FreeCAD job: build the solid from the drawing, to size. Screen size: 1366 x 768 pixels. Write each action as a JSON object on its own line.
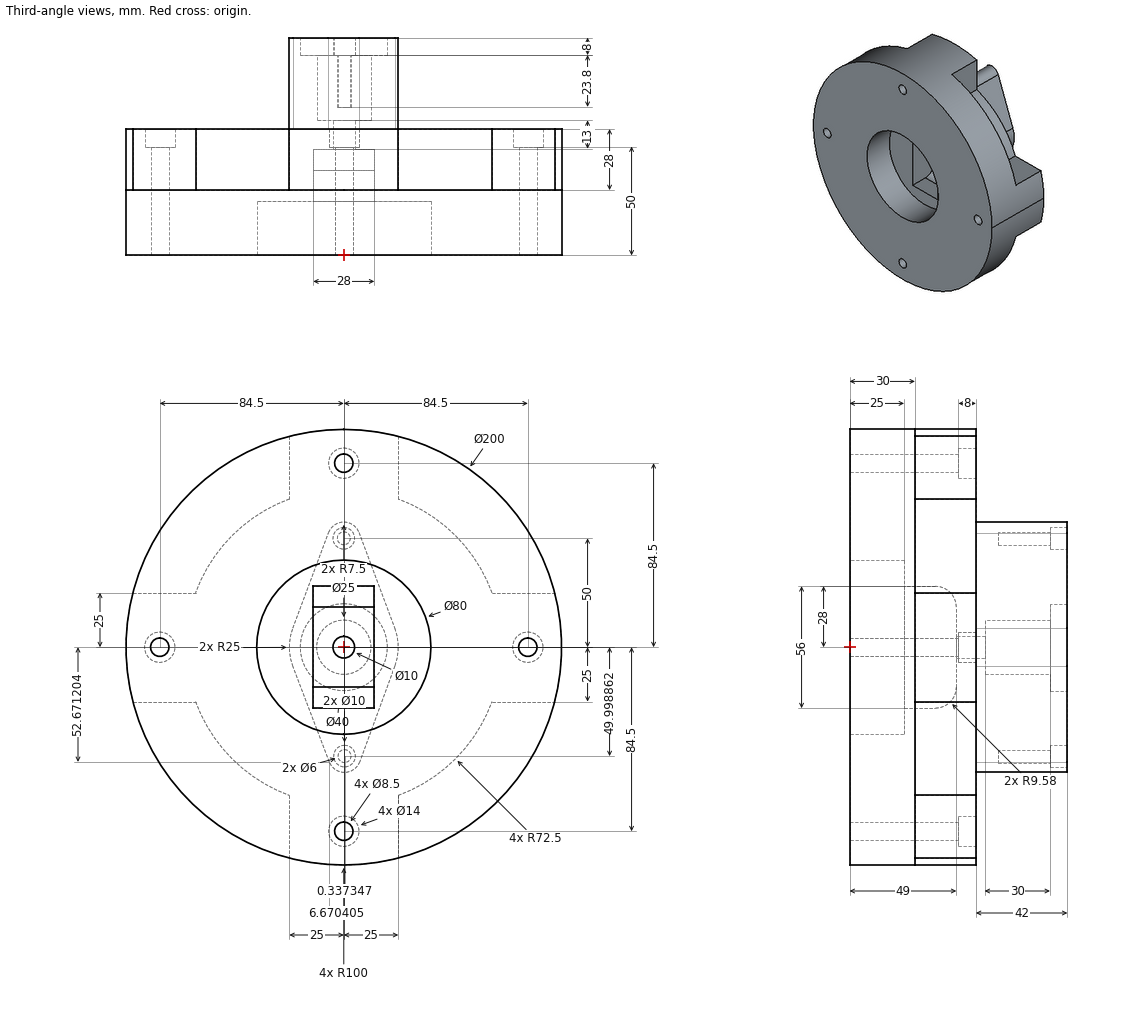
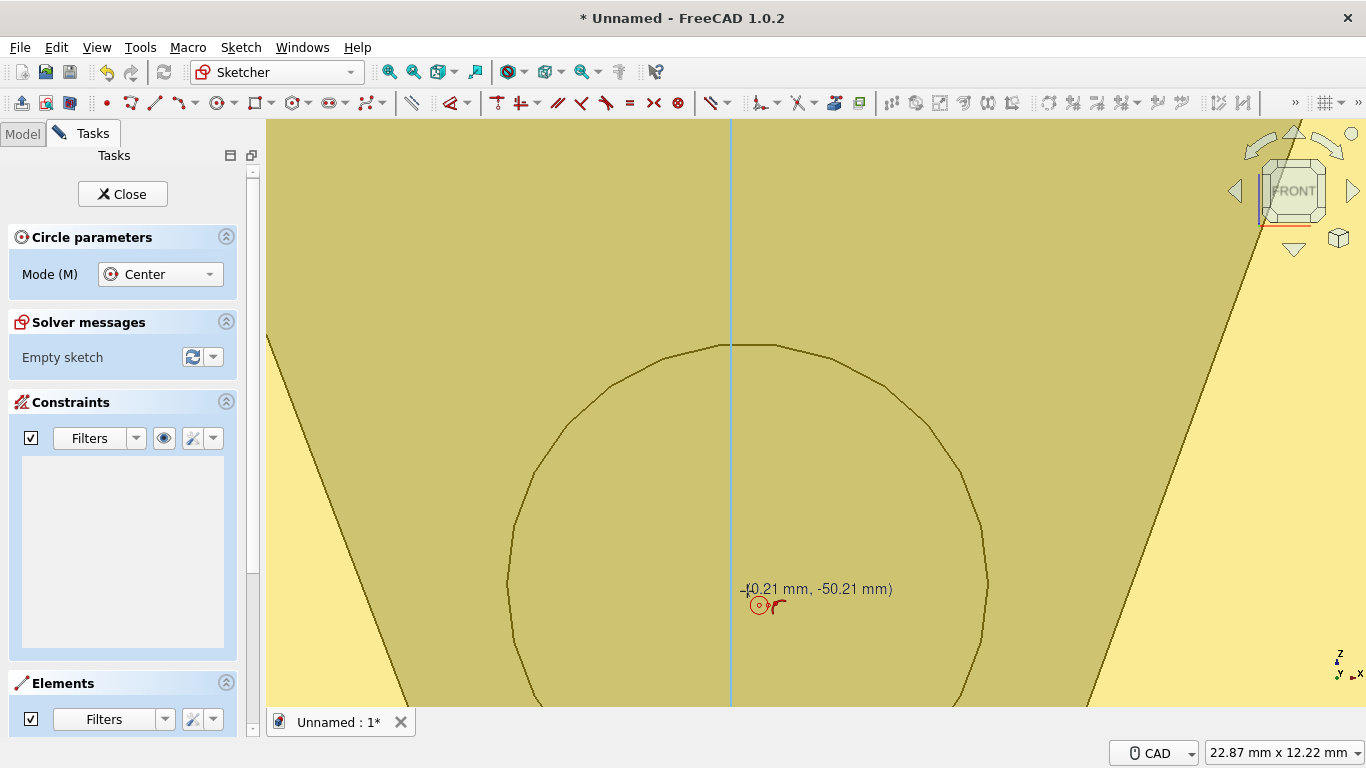
{"action": "left_click", "coordinate": [748, 584]}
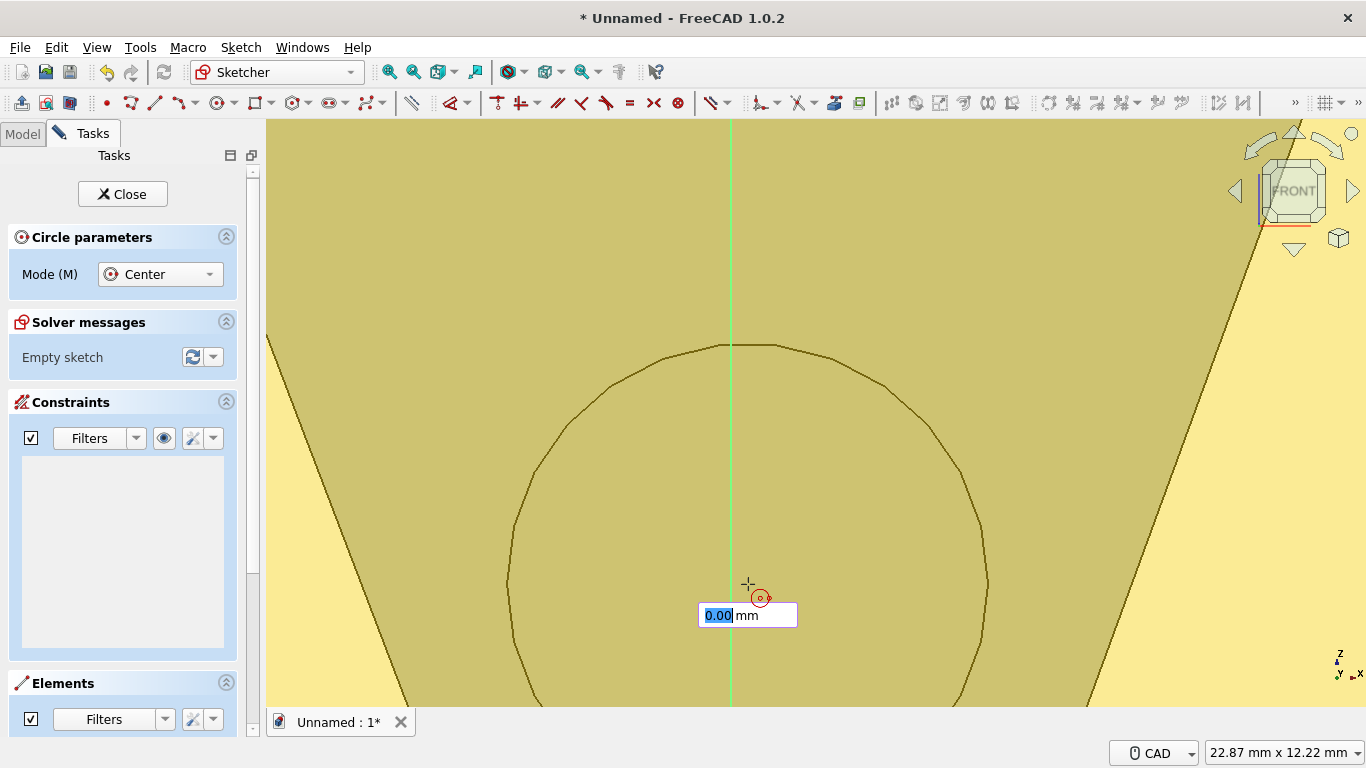
{"action": "scroll", "coordinate": [748, 592], "scroll_direction": "down", "scroll_amount": 13}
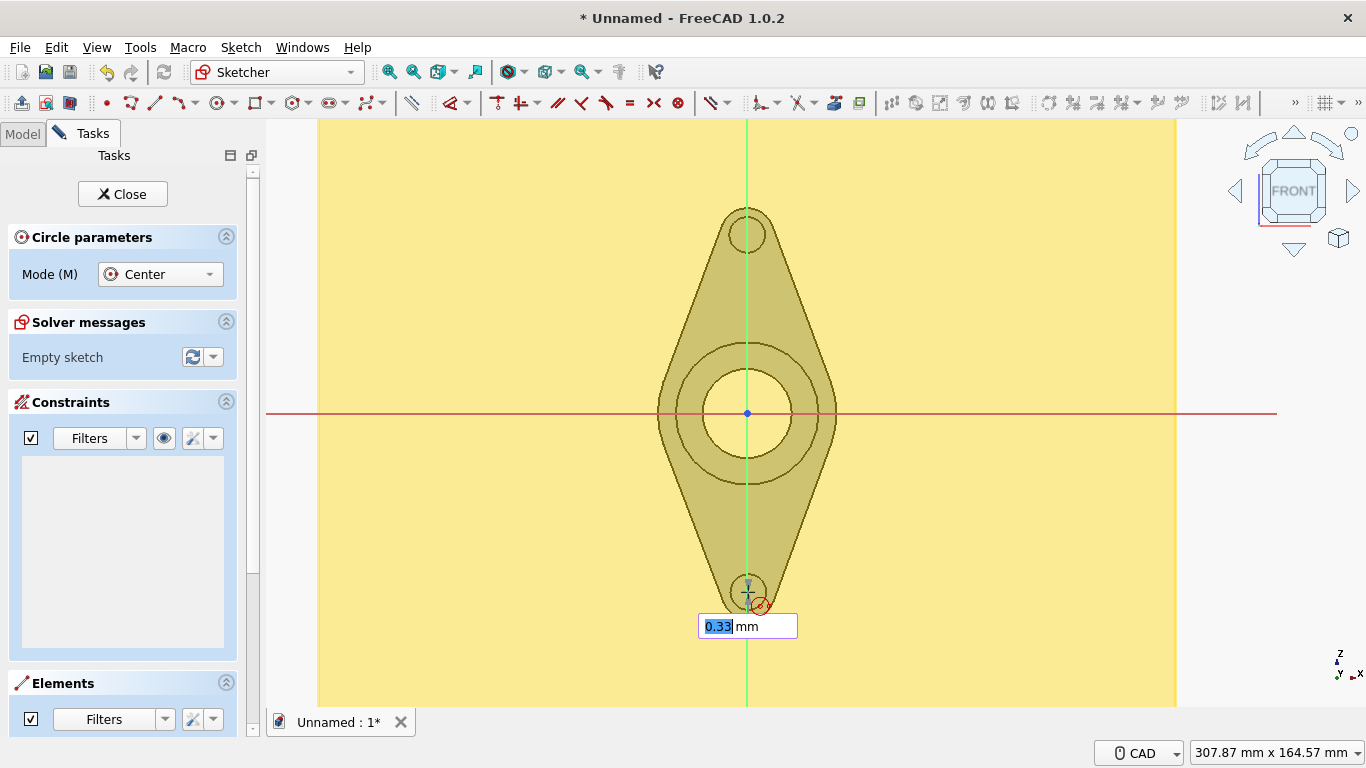
{"action": "scroll", "coordinate": [756, 585], "scroll_direction": "up", "scroll_amount": 3}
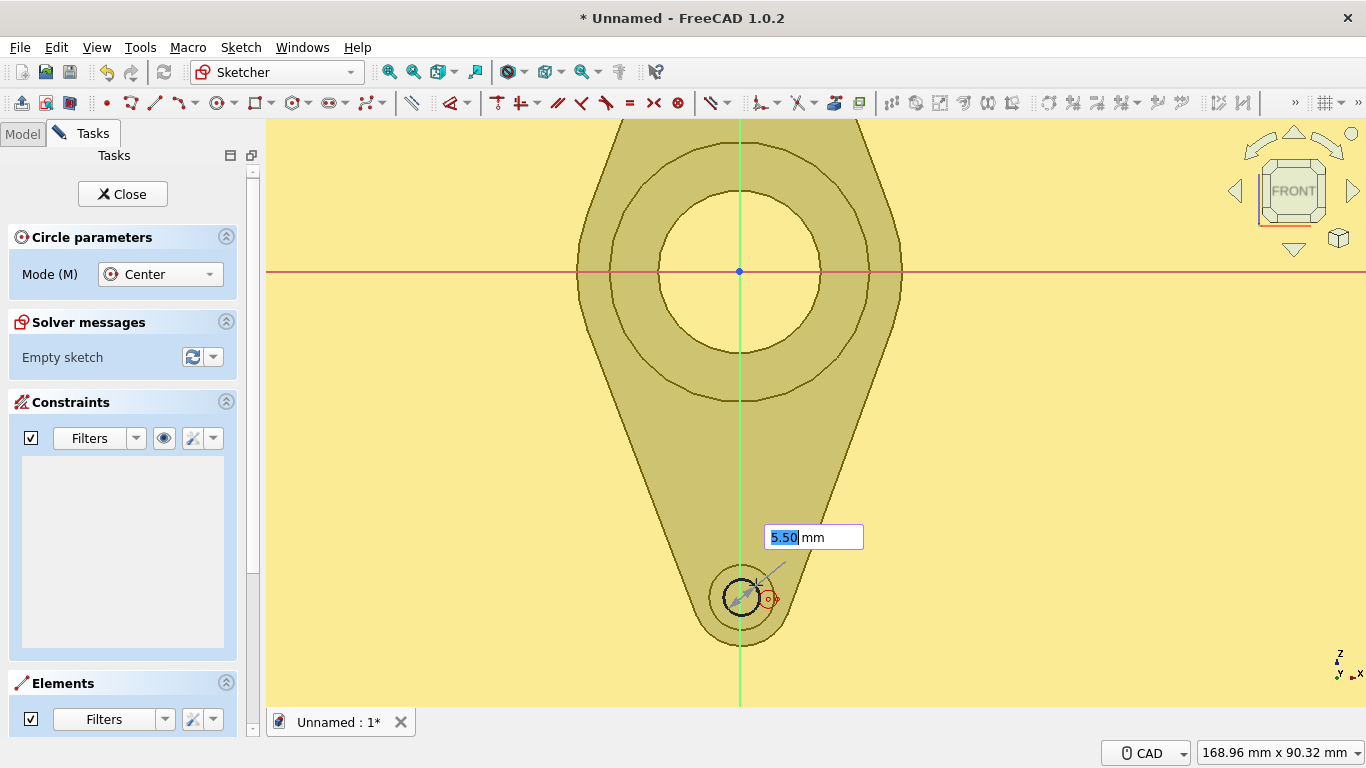
{"action": "left_click", "coordinate": [756, 584]}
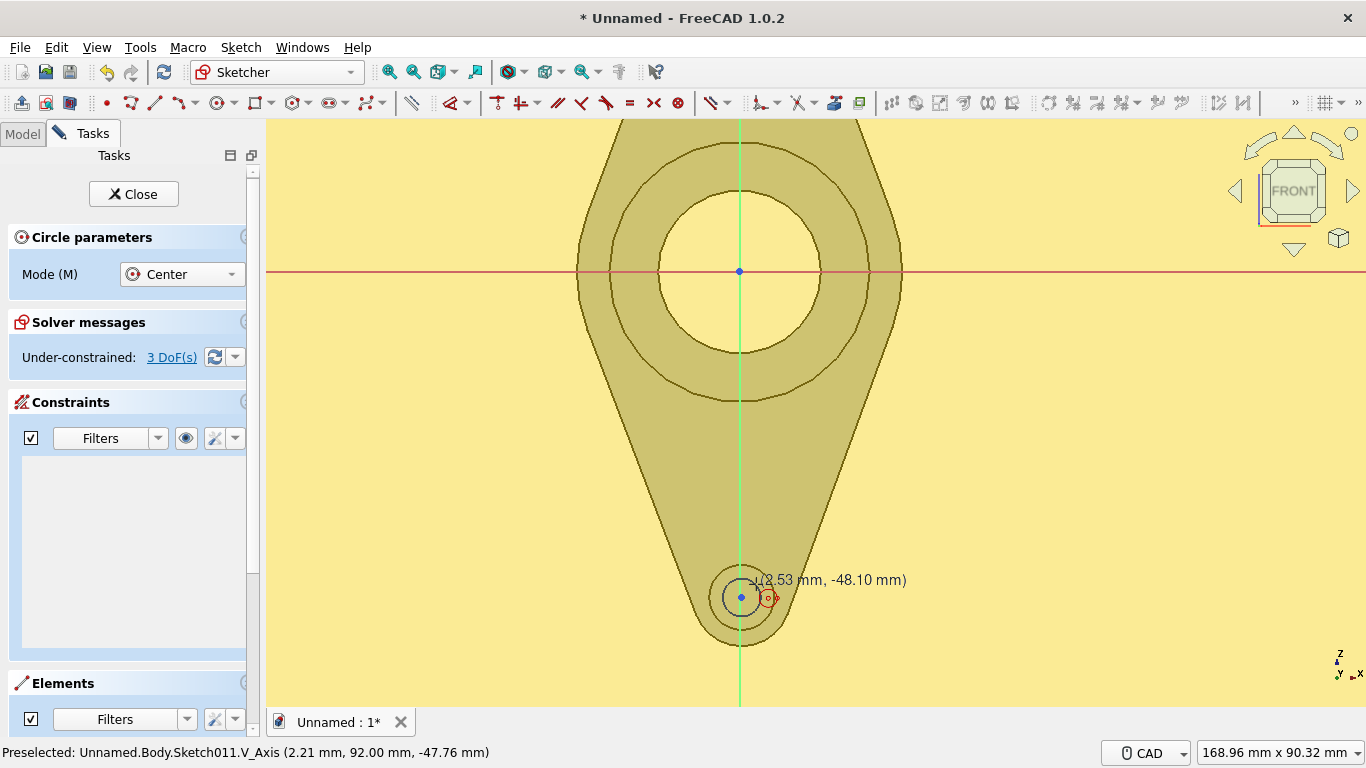
{"action": "scroll", "coordinate": [756, 585], "scroll_direction": "down", "scroll_amount": 3}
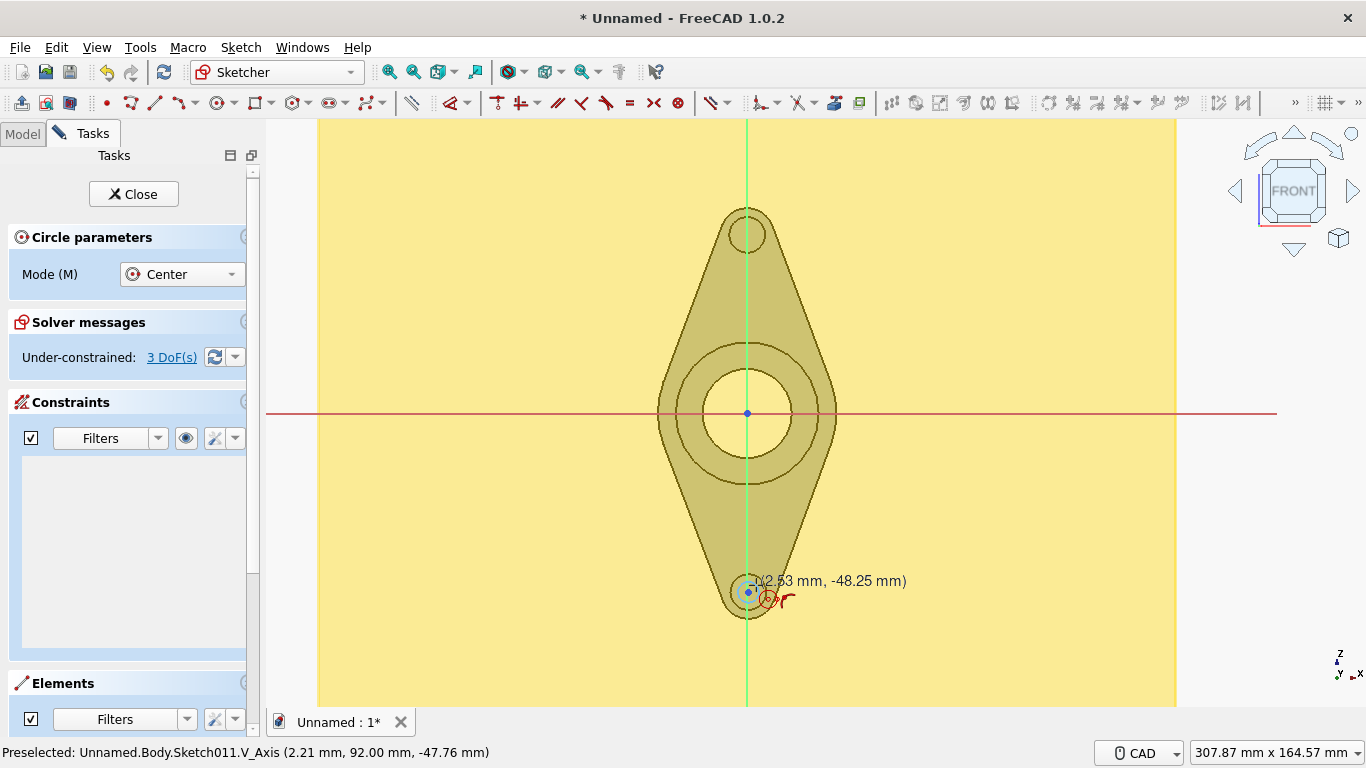
{"action": "scroll", "coordinate": [747, 235], "scroll_direction": "up", "scroll_amount": 4}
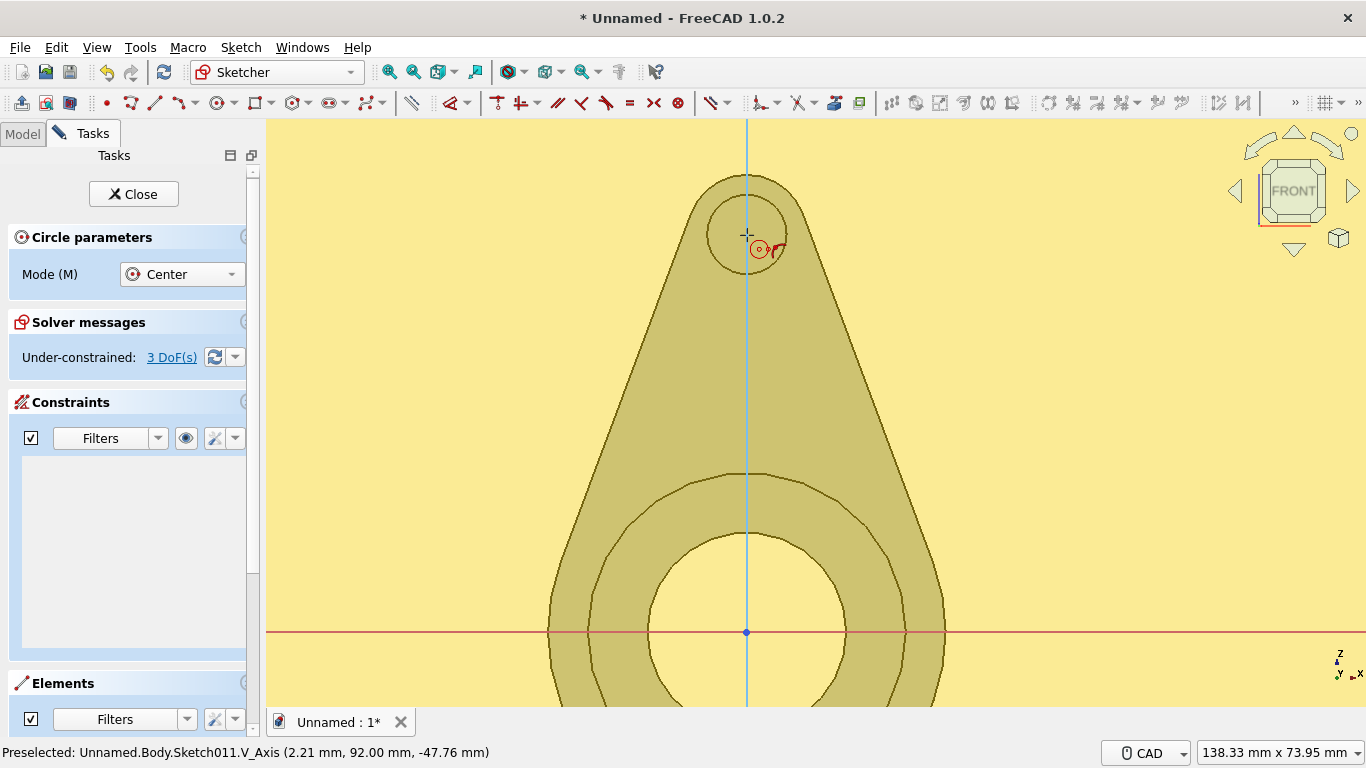
{"action": "left_click", "coordinate": [747, 234]}
{"action": "left_click", "coordinate": [764, 218]}
{"action": "key", "text": "Escape"}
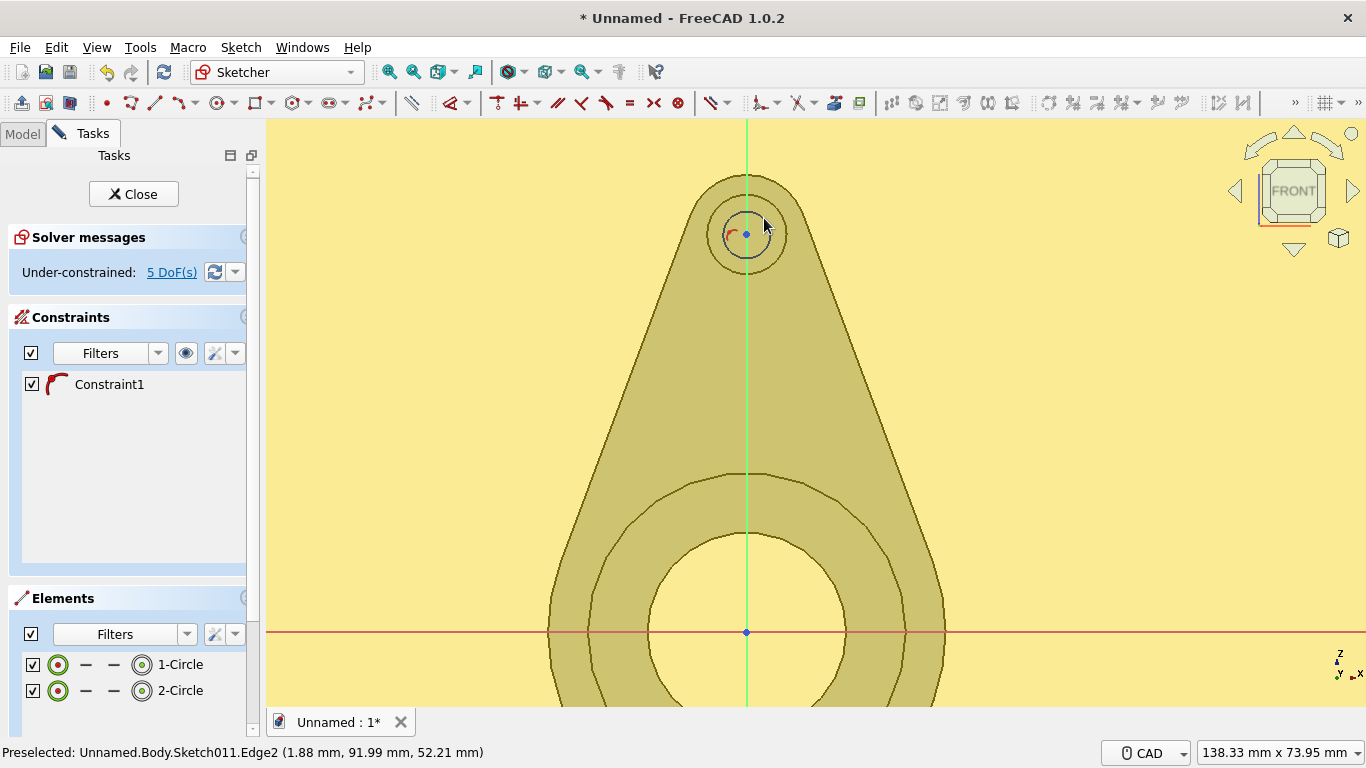
{"action": "scroll", "coordinate": [747, 234], "scroll_direction": "down", "scroll_amount": 4}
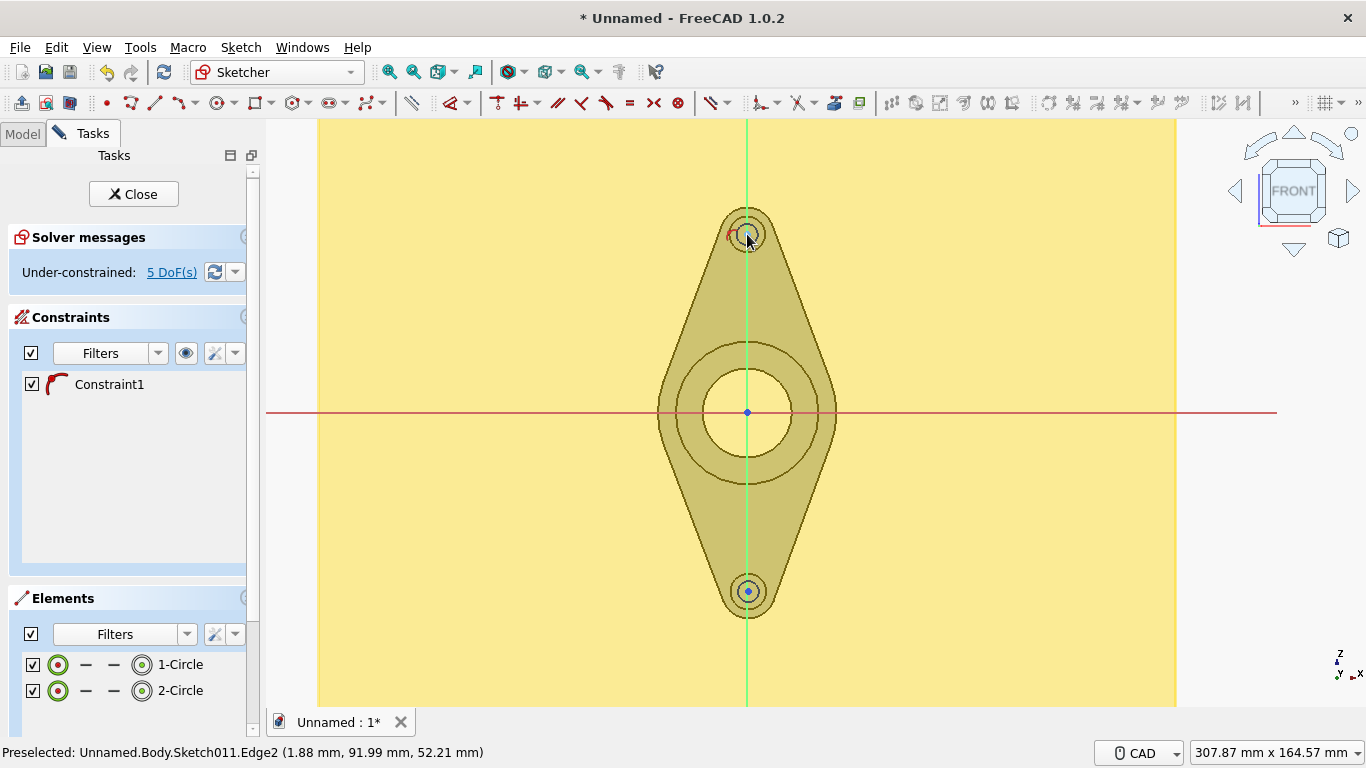
{"action": "scroll", "coordinate": [756, 584], "scroll_direction": "up", "scroll_amount": 3}